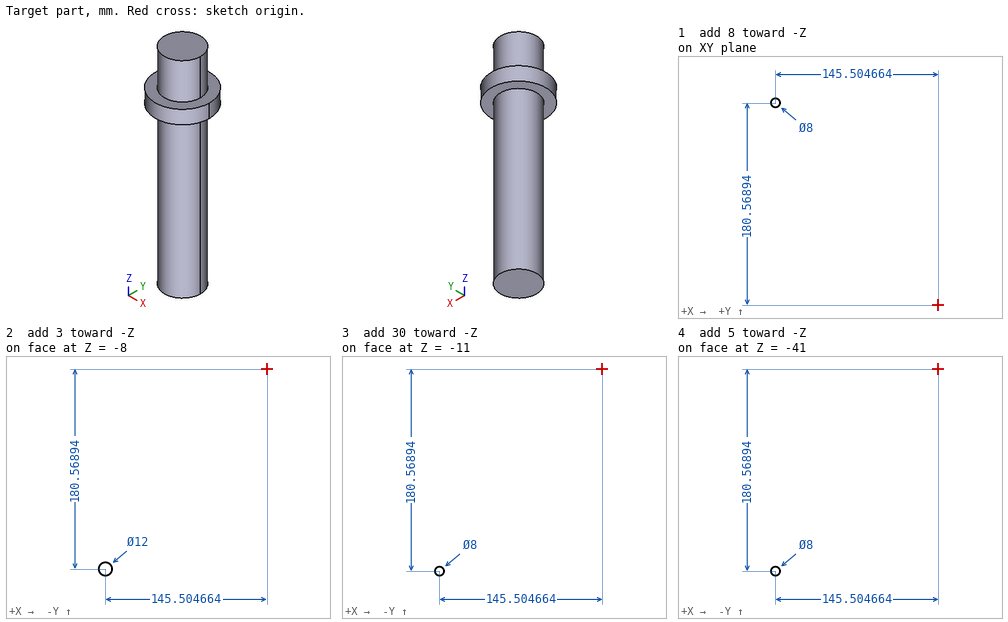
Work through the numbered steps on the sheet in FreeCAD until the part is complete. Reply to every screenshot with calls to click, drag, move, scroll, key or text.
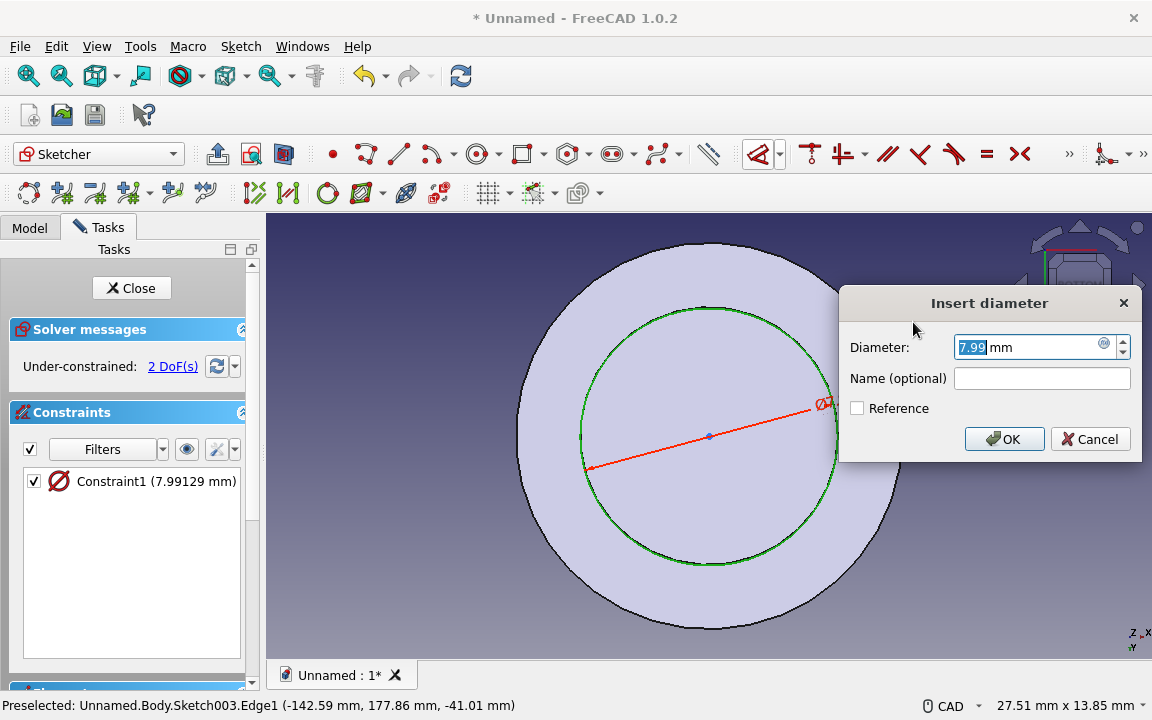
text(8)
key(Return)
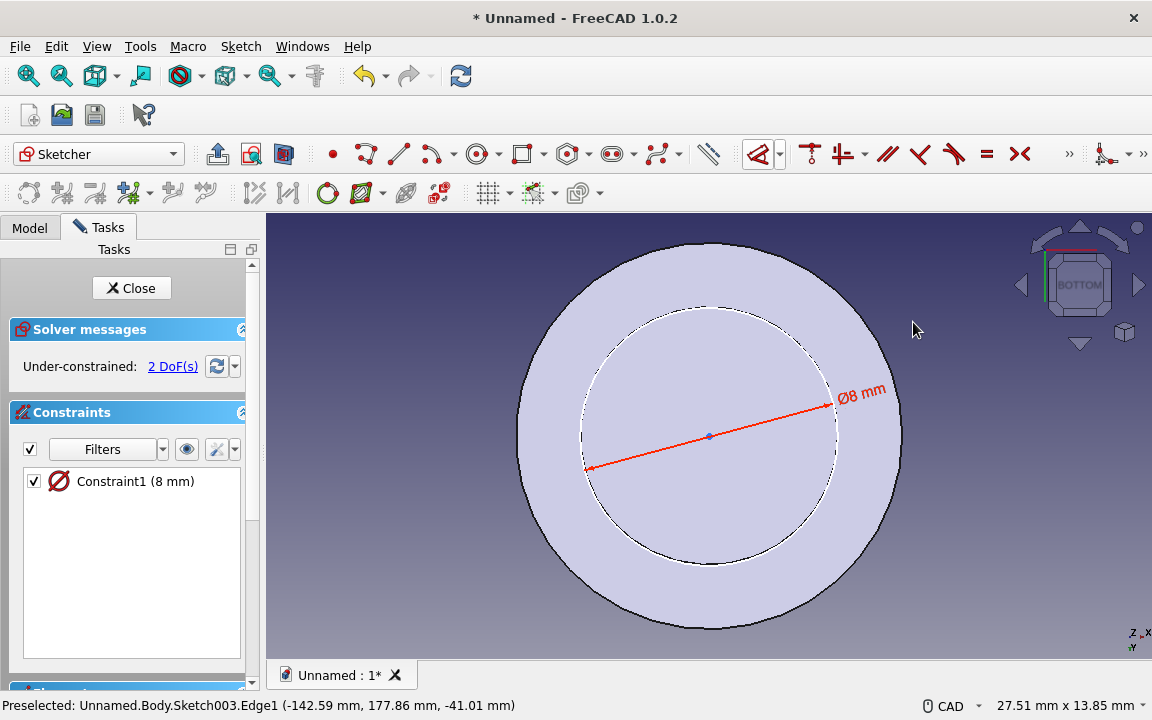
click(709, 437)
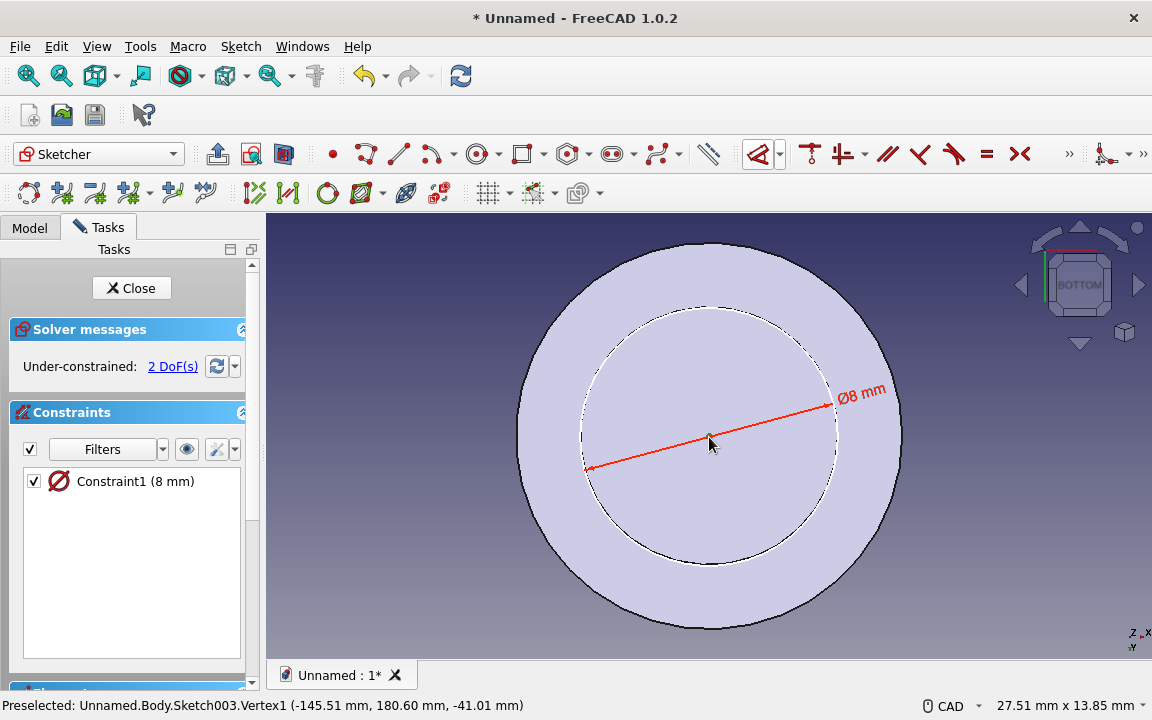
click(780, 154)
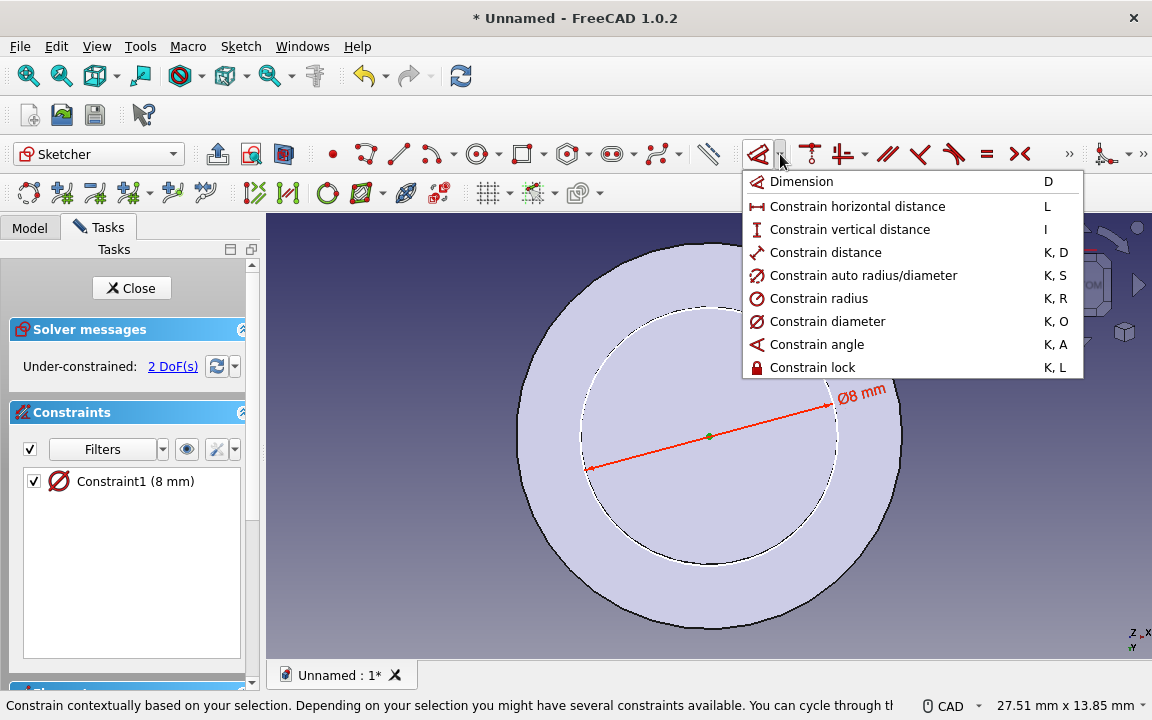
click(913, 230)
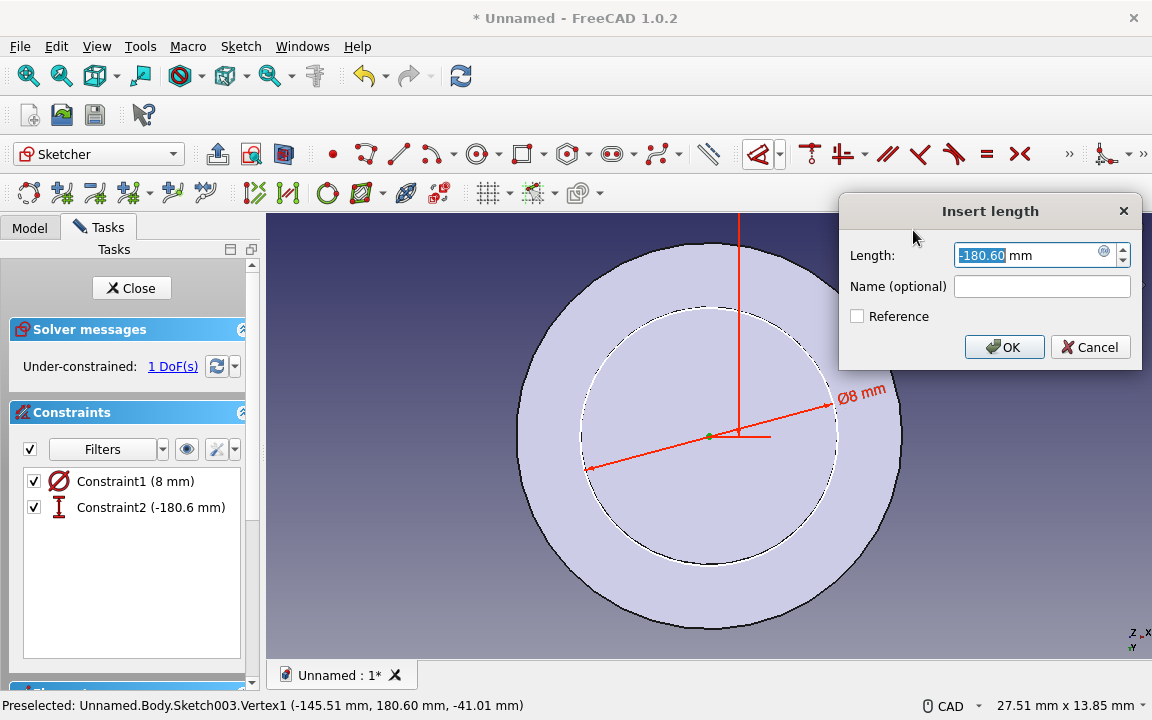
text(-180.56894)
key(Return)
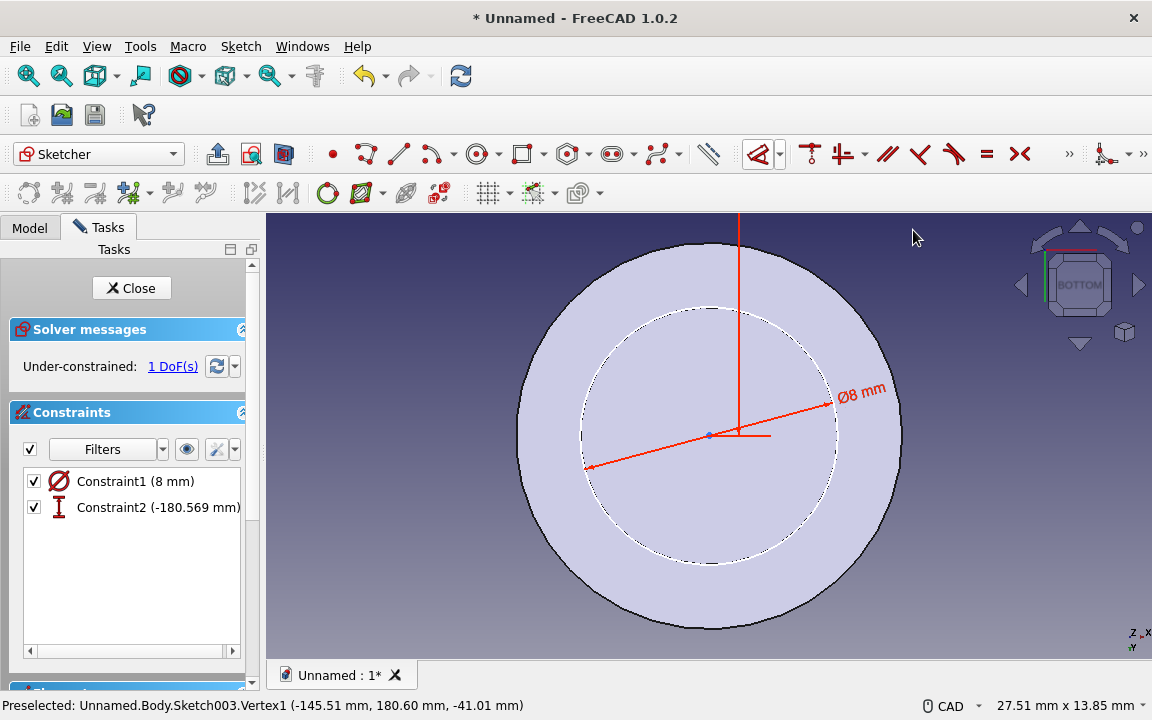
click(709, 436)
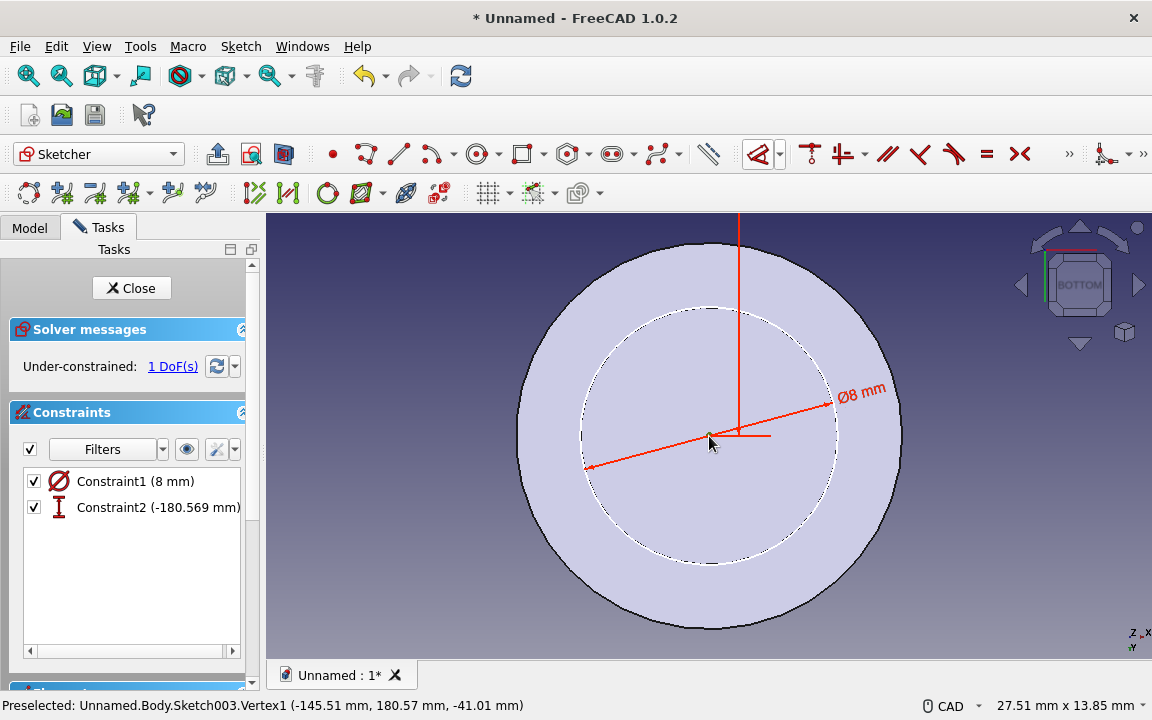
key(l)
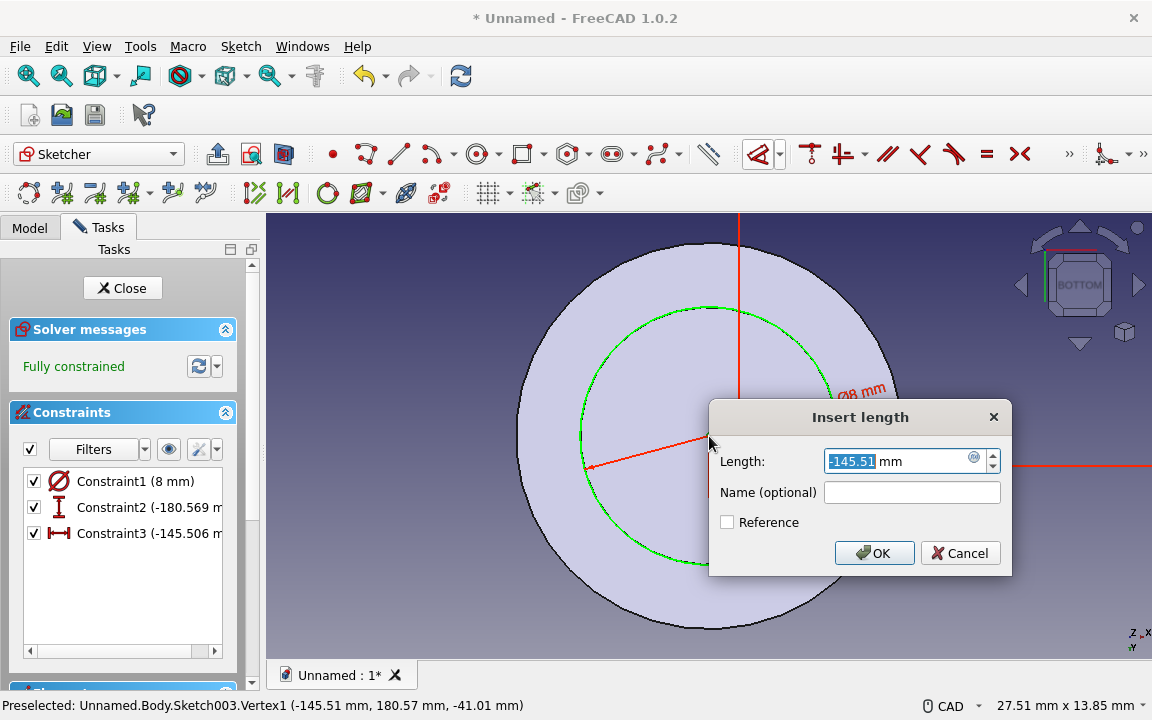
text(-145.504664)
key(Return)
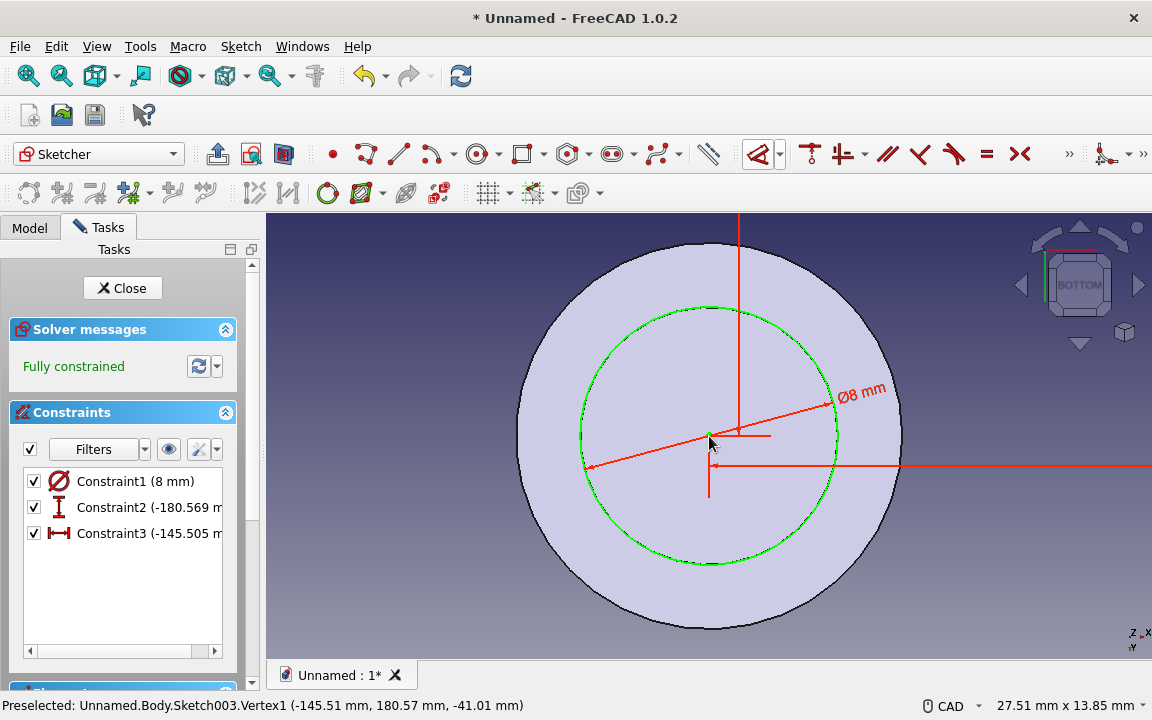
click(123, 288)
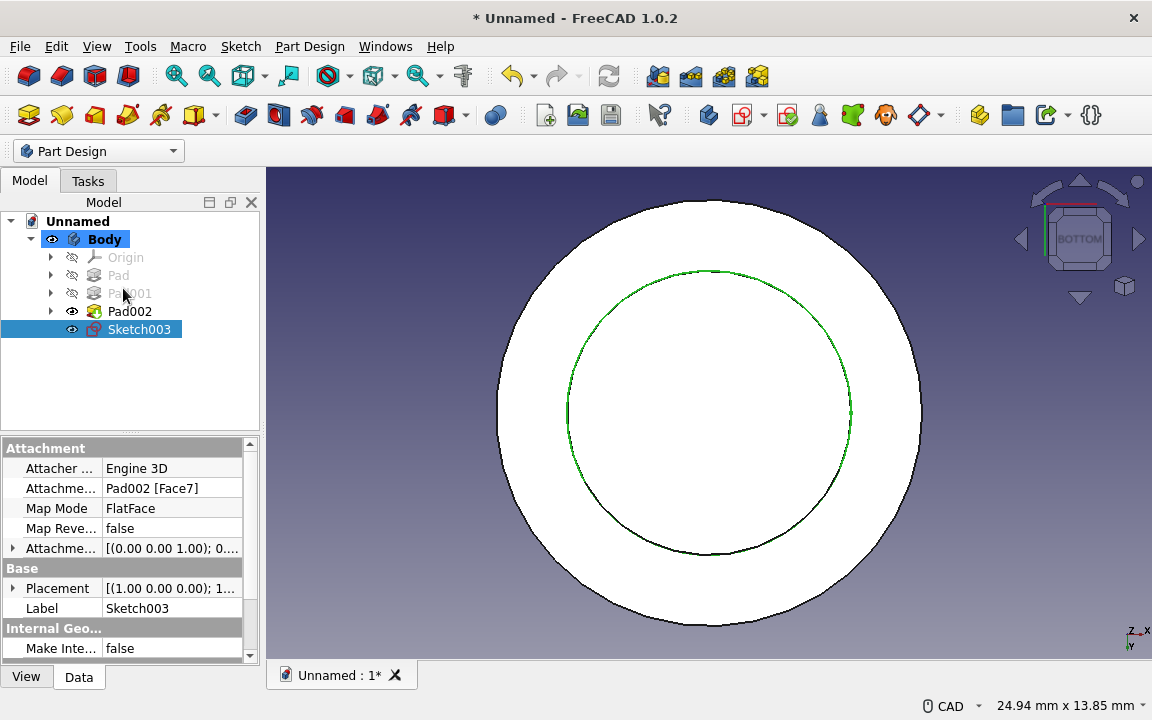
click(29, 116)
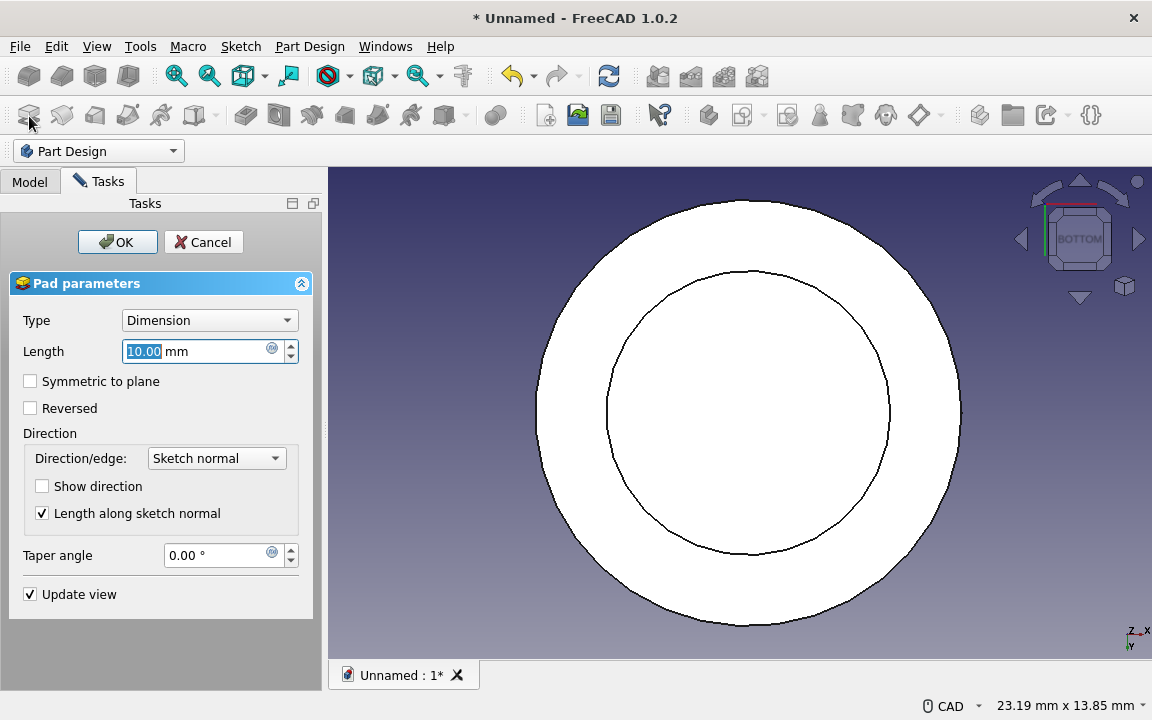
text(5)
key(Tab)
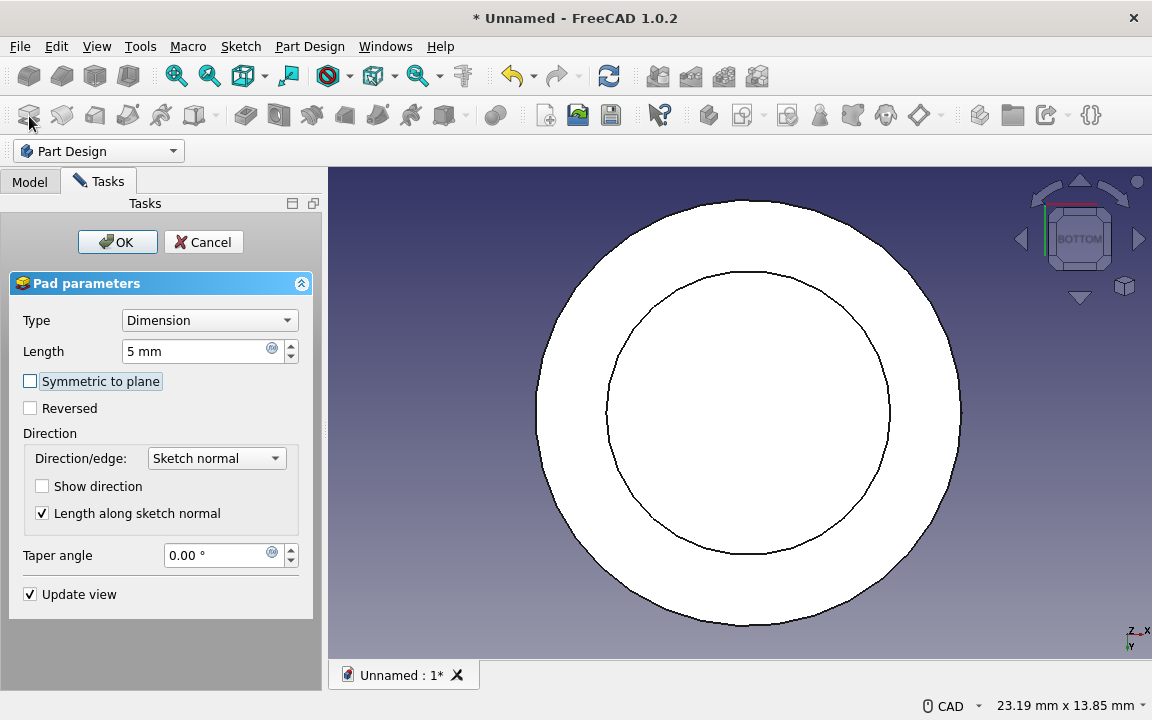
click(118, 242)